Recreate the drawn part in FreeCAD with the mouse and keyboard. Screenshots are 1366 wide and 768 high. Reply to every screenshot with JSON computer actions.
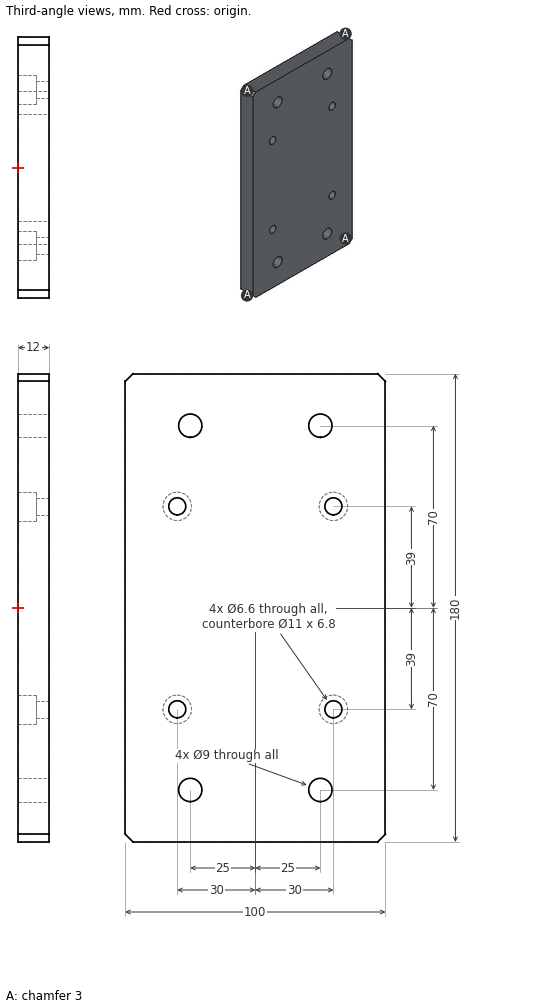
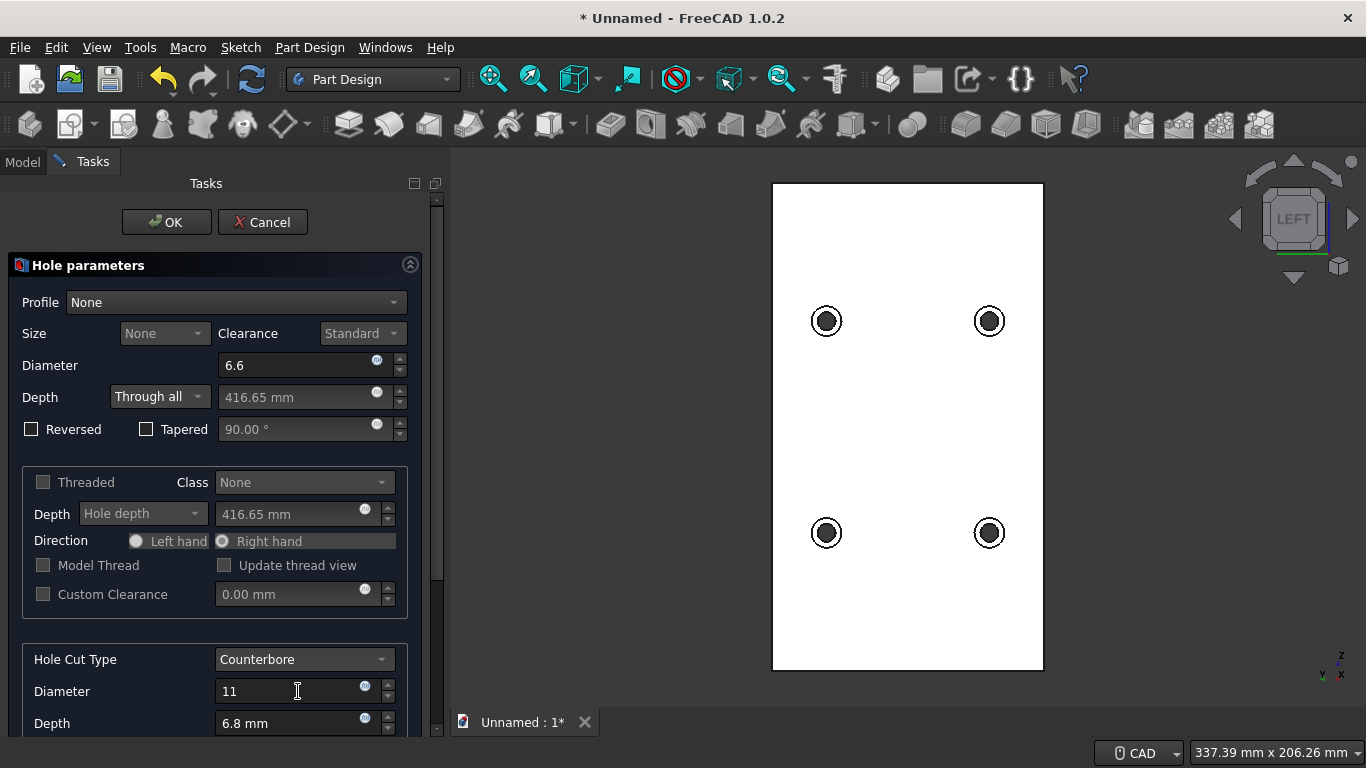
{"action": "left_click", "coordinate": [167, 222]}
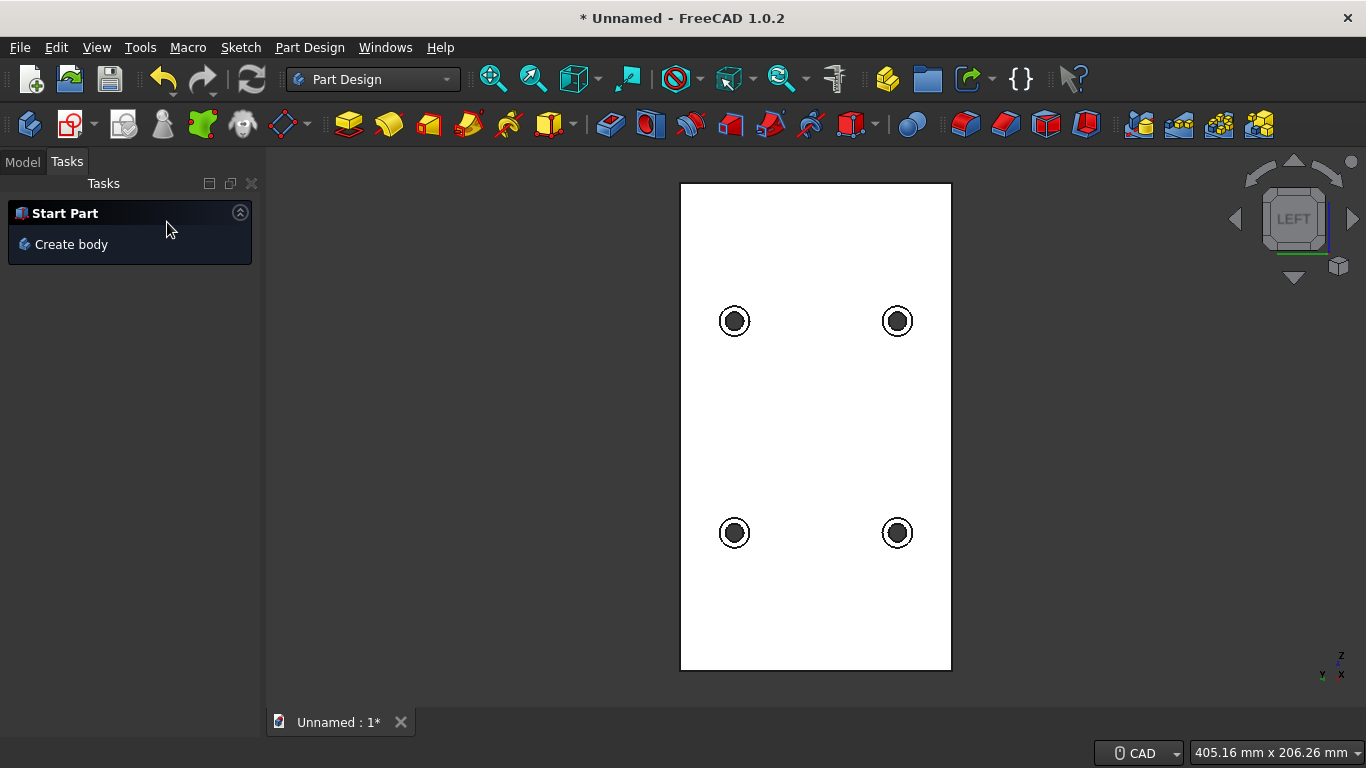
{"action": "left_click", "coordinate": [816, 426]}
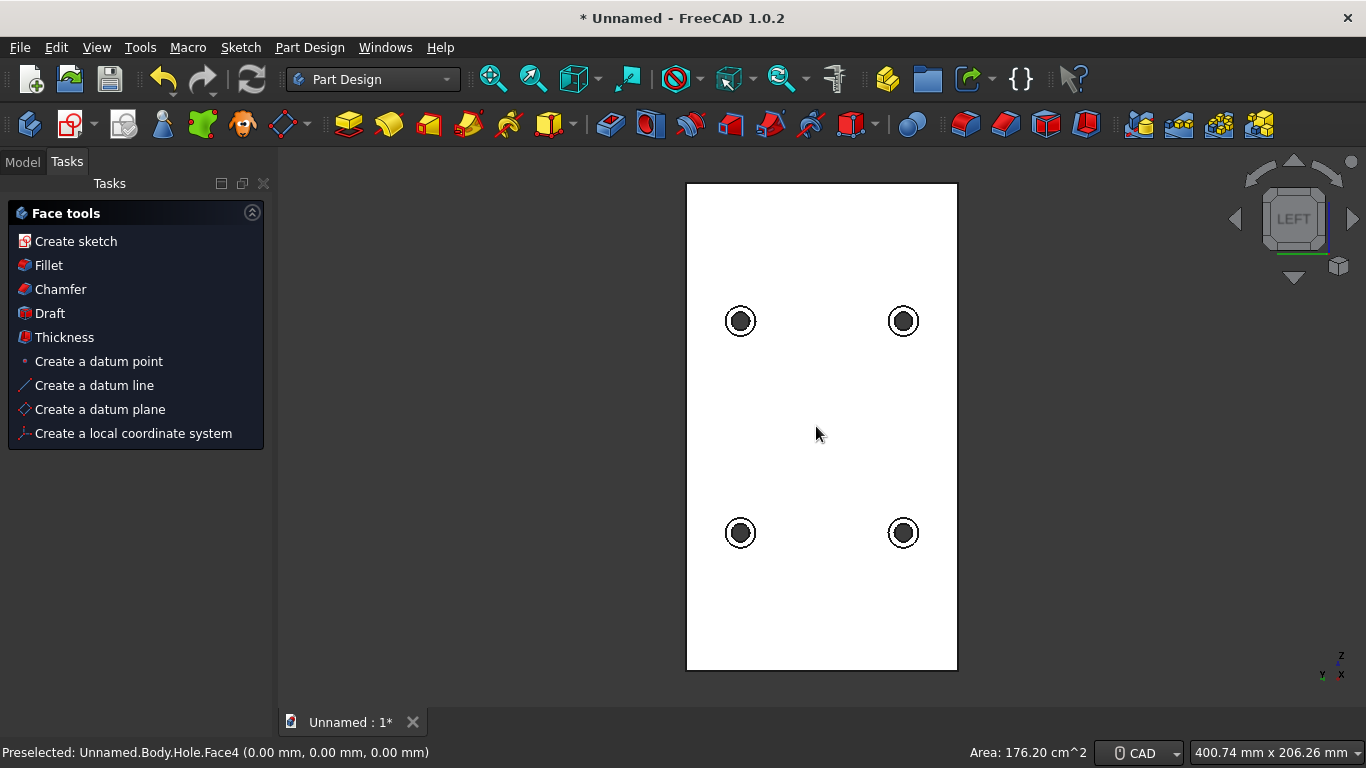
{"action": "left_click", "coordinate": [70, 124]}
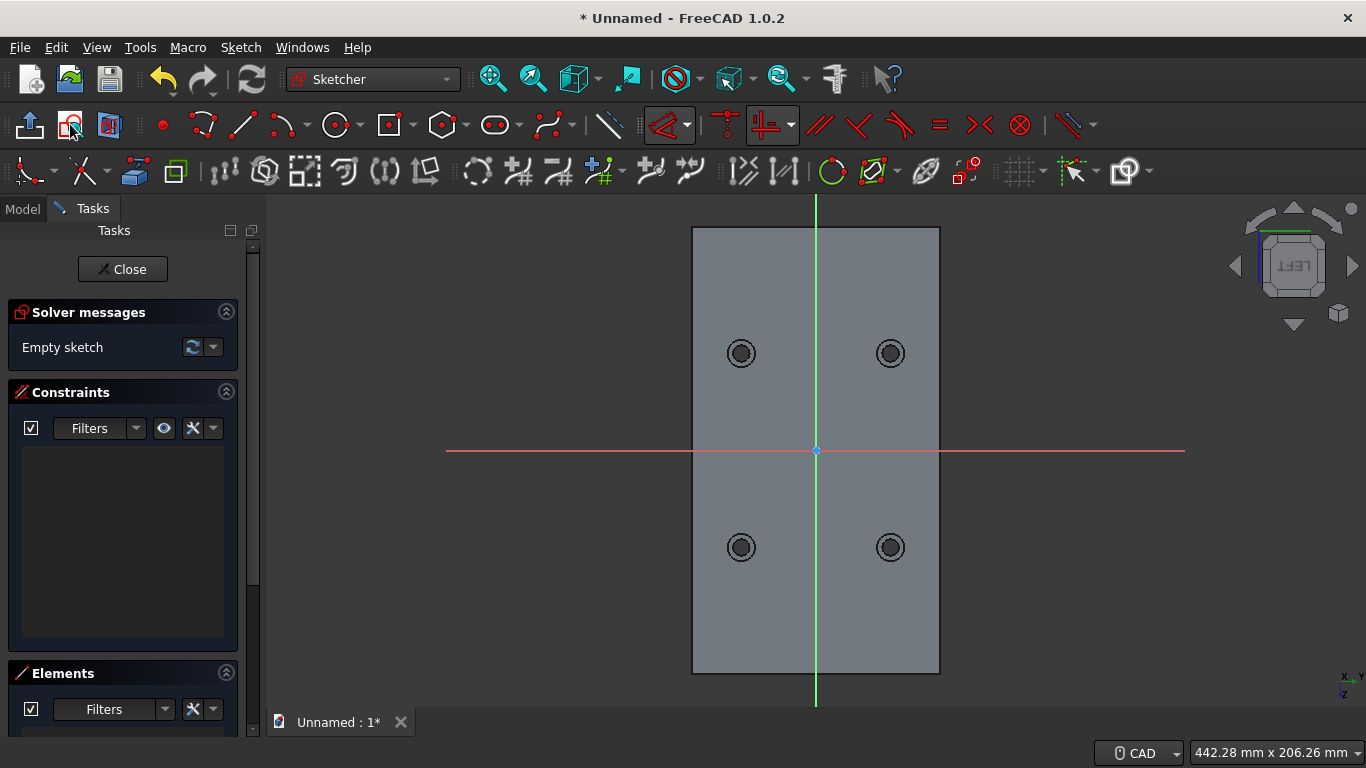
{"action": "left_click", "coordinate": [336, 126]}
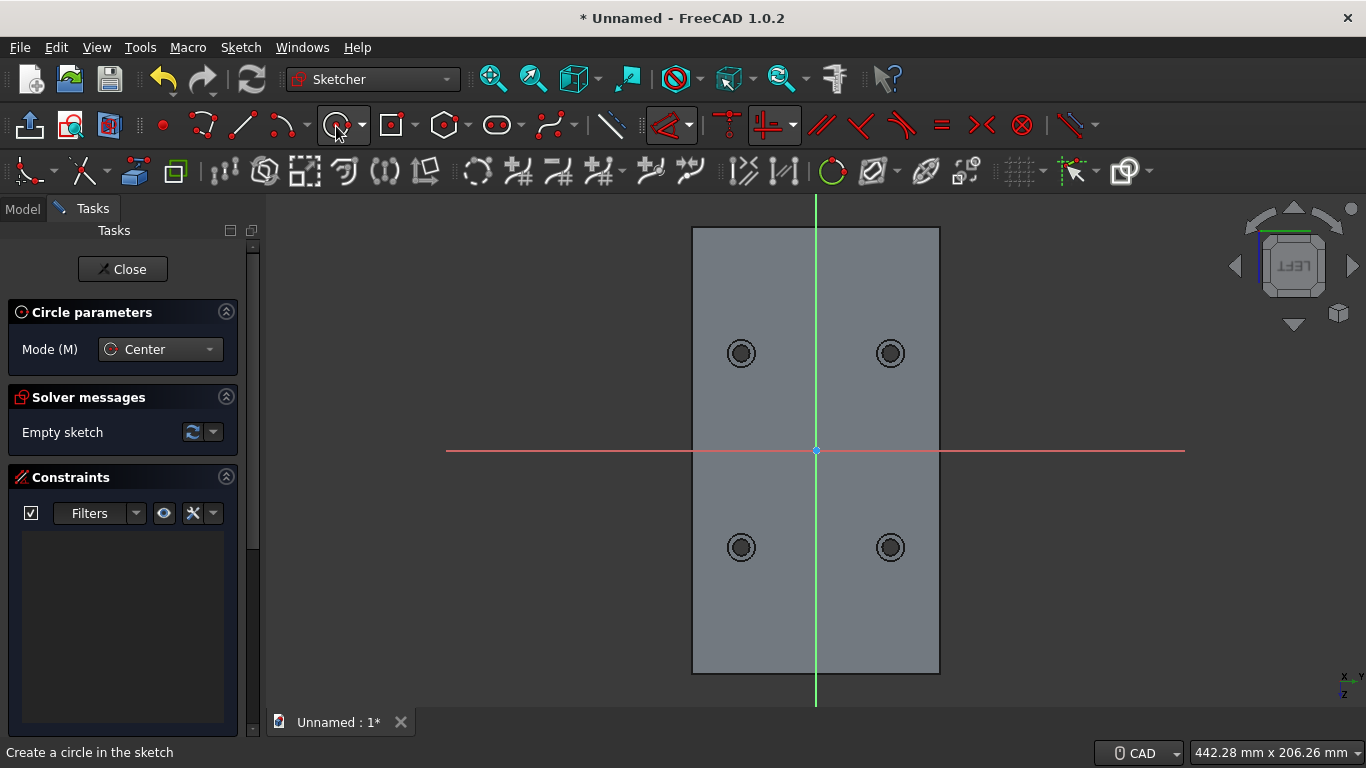
{"action": "scroll", "coordinate": [878, 276], "scroll_direction": "up", "scroll_amount": 4}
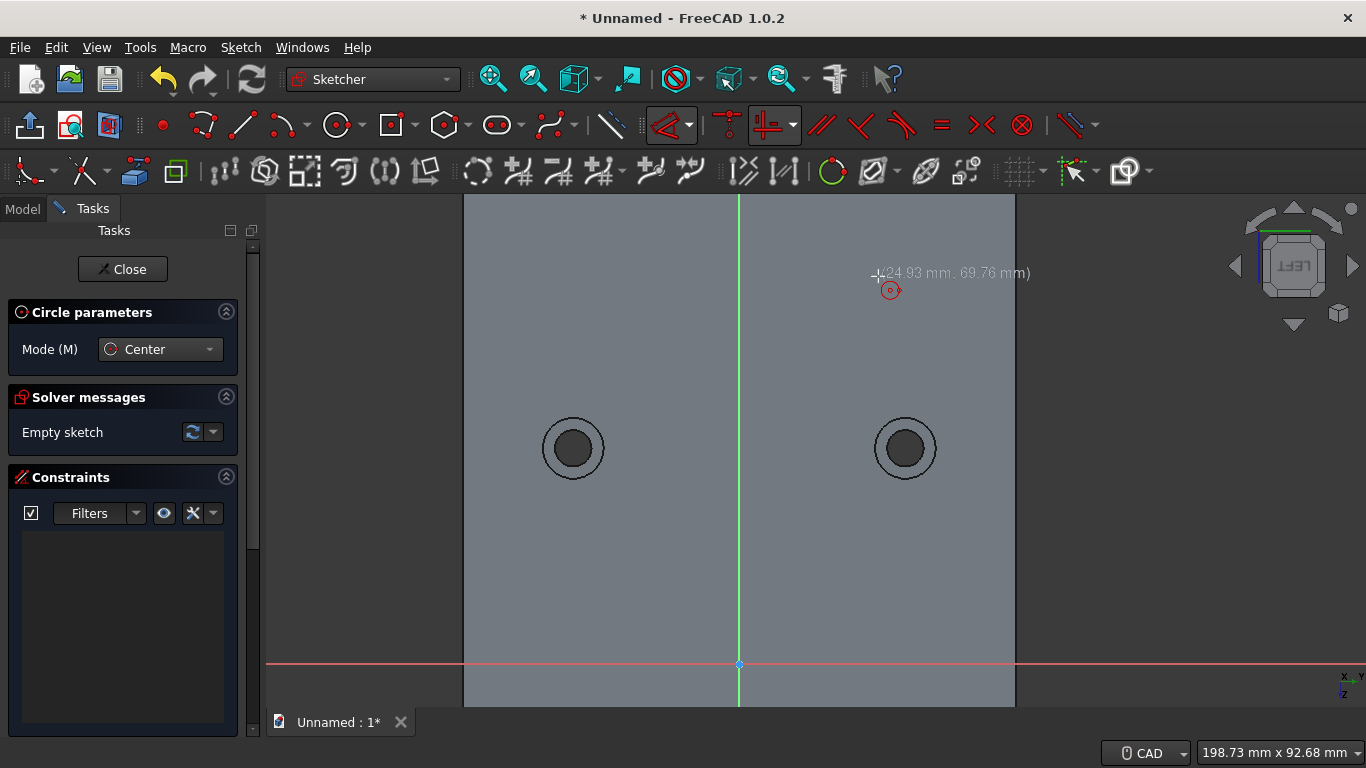
{"action": "left_click", "coordinate": [878, 277]}
{"action": "left_click", "coordinate": [895, 259]}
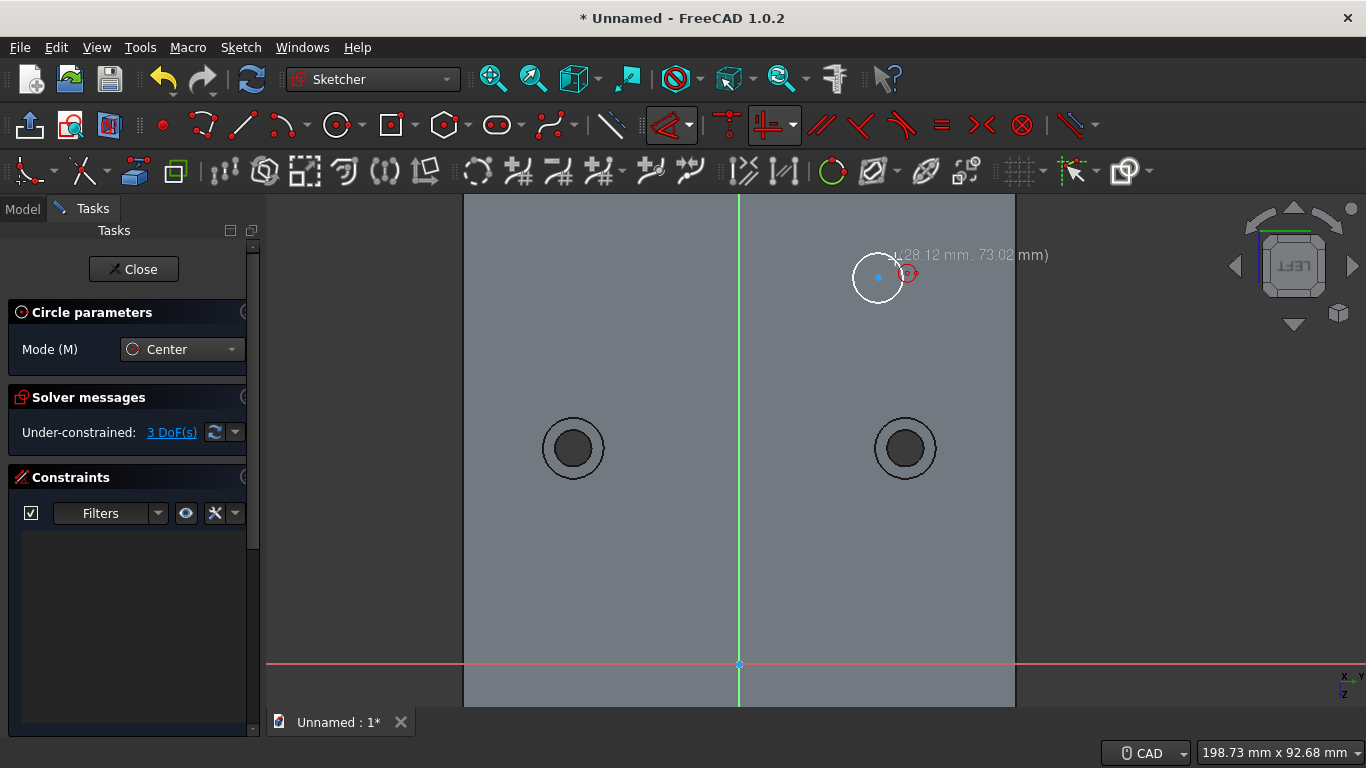
{"action": "left_click", "coordinate": [601, 277]}
{"action": "left_click", "coordinate": [619, 259]}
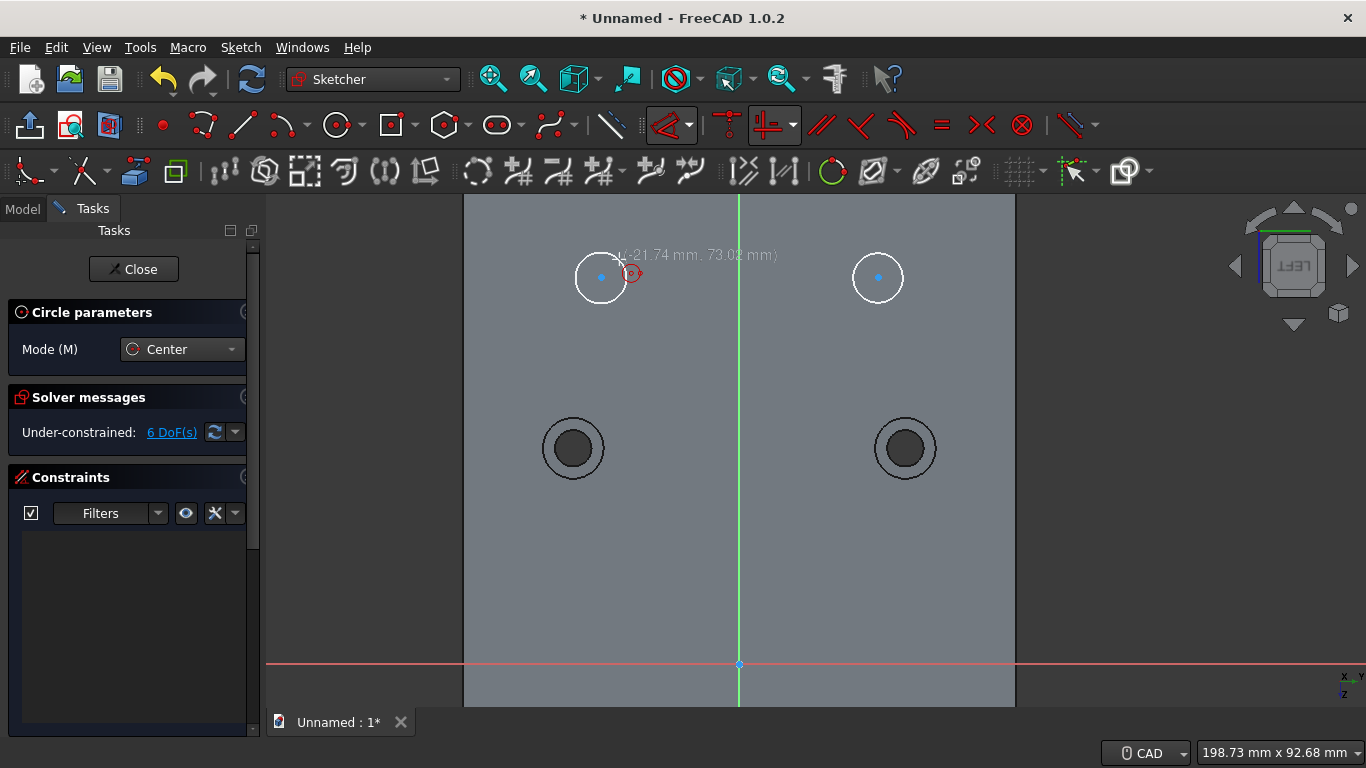
{"action": "scroll", "coordinate": [752, 326], "scroll_direction": "down", "scroll_amount": 5}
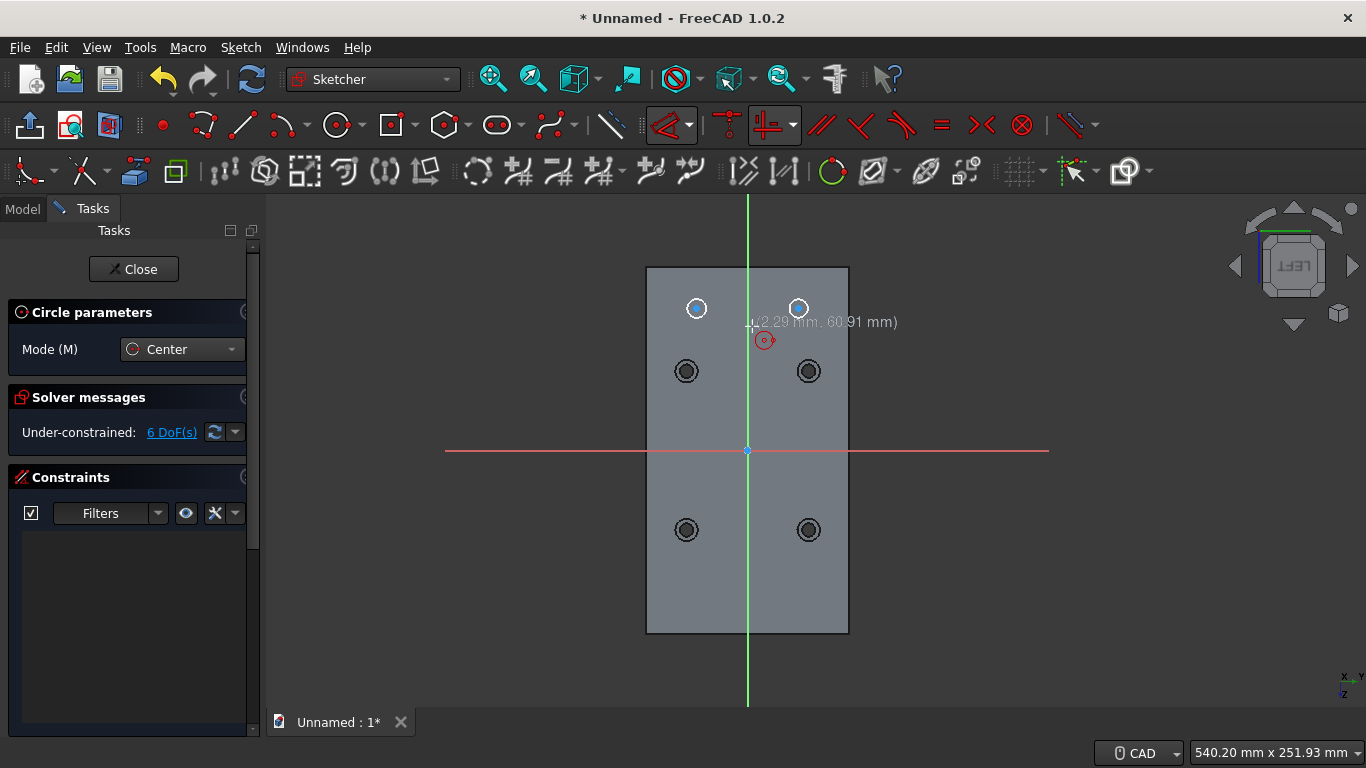
{"action": "scroll", "coordinate": [799, 593], "scroll_direction": "up", "scroll_amount": 5}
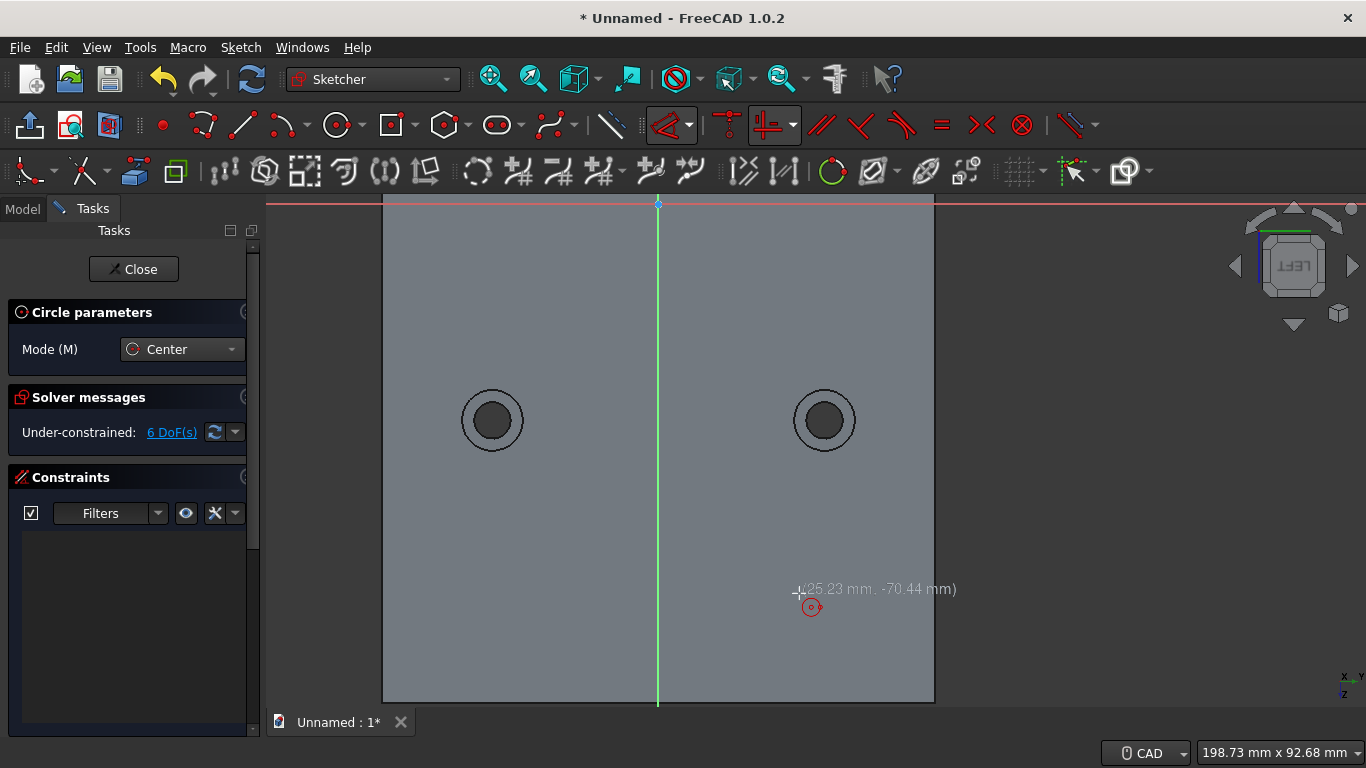
{"action": "left_click", "coordinate": [797, 592]}
{"action": "left_click", "coordinate": [814, 574]}